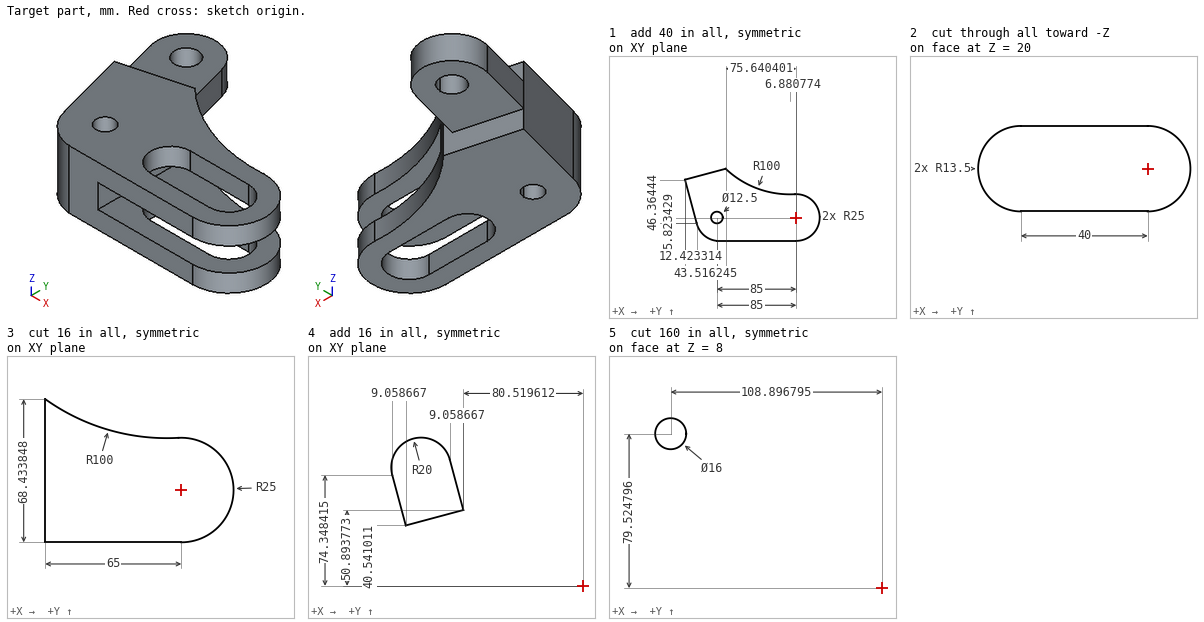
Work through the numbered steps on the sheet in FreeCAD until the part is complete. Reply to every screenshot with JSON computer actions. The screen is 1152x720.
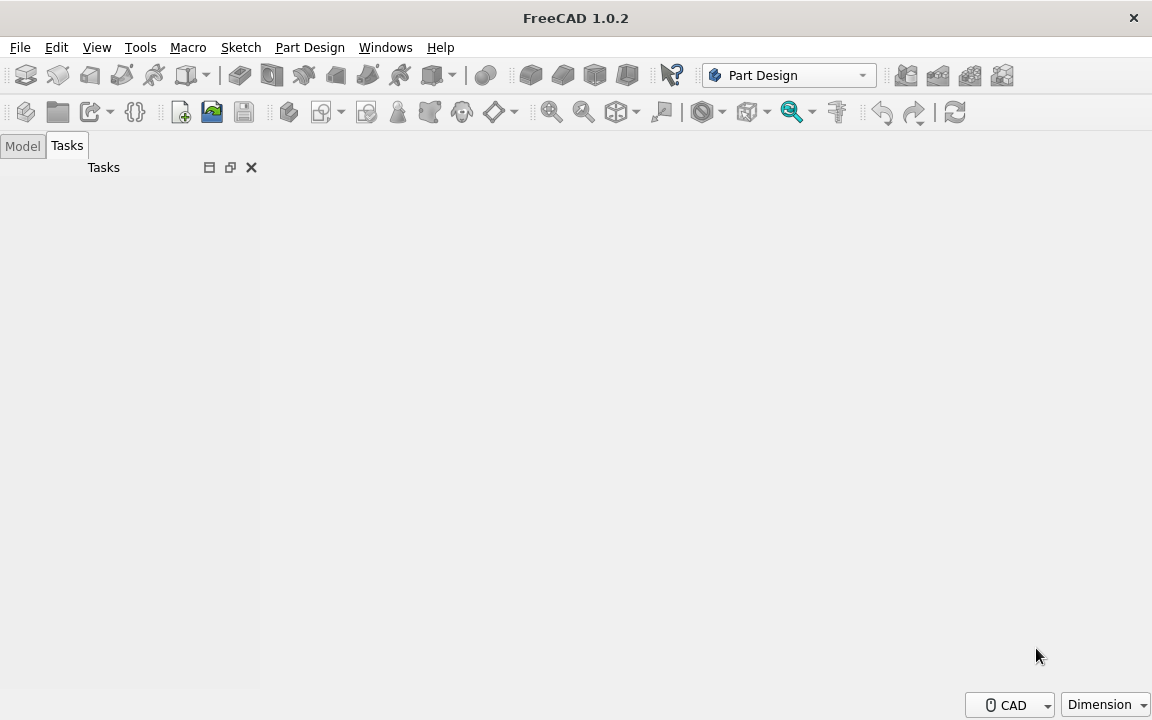
{"action": "left_click", "coordinate": [180, 112]}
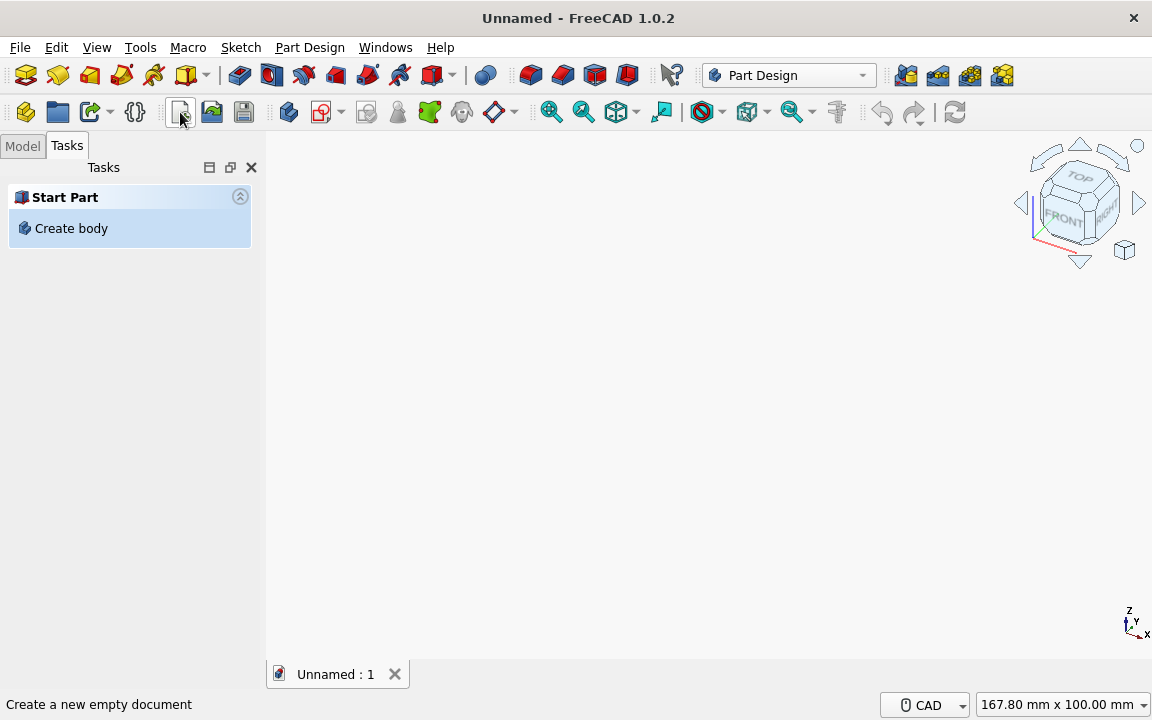
{"action": "left_click", "coordinate": [322, 112]}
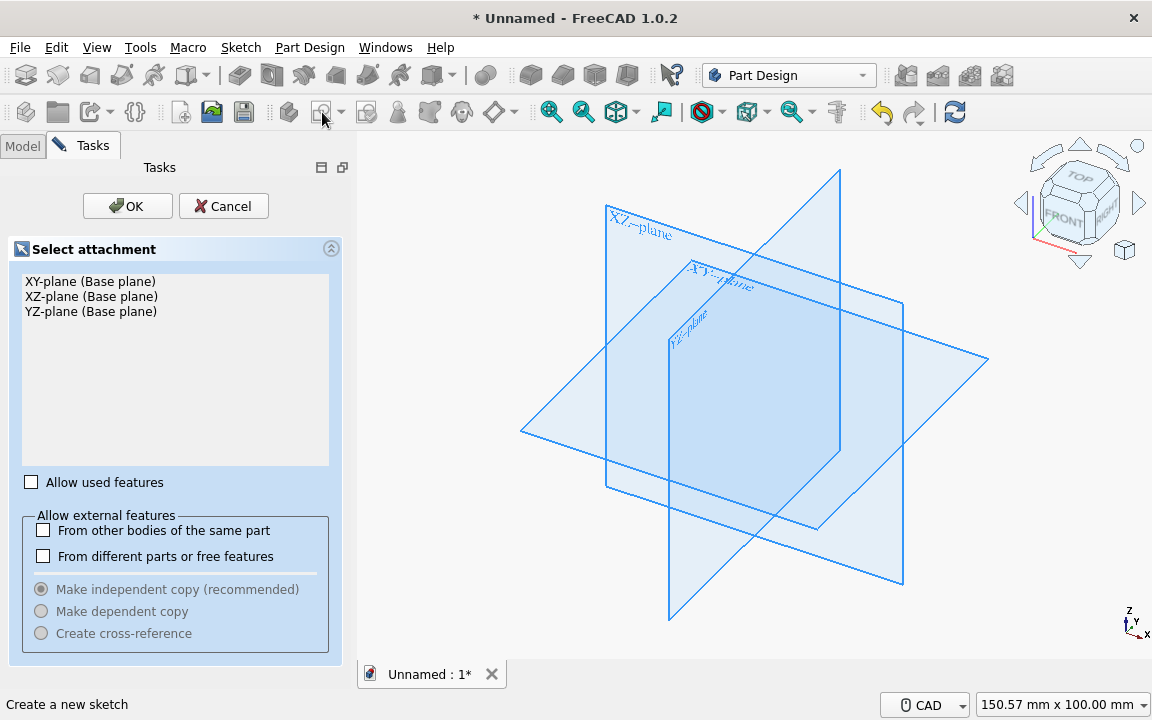
{"action": "left_click", "coordinate": [82, 282]}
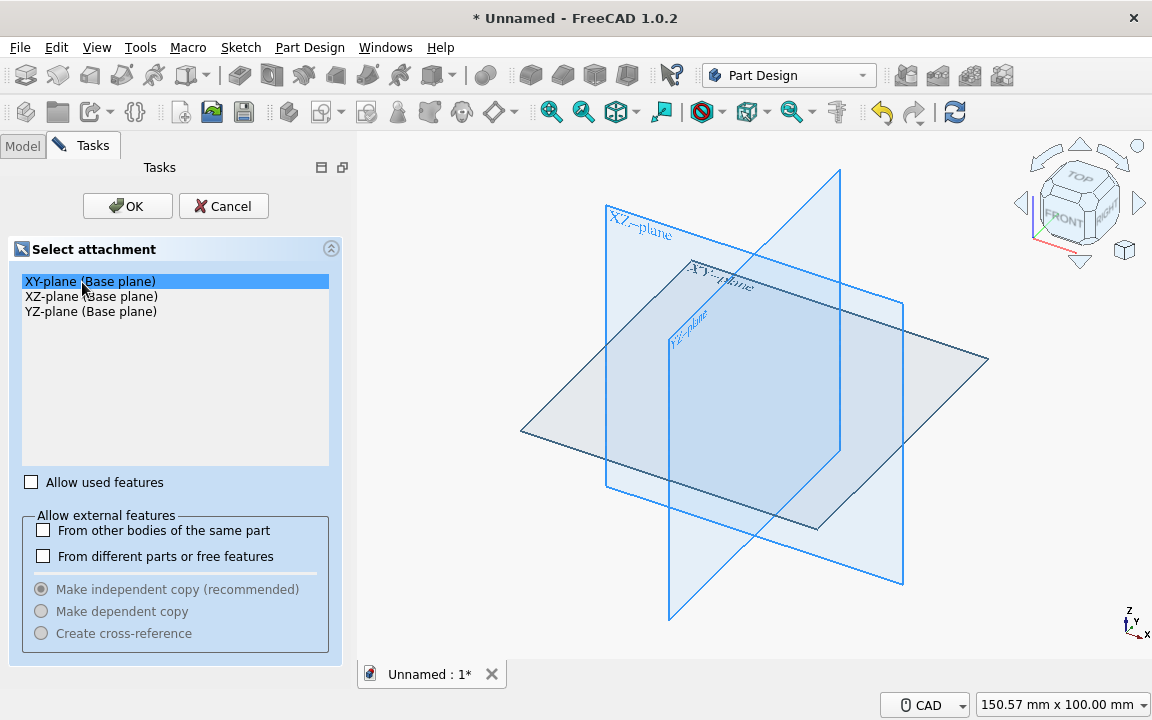
{"action": "left_click", "coordinate": [128, 206]}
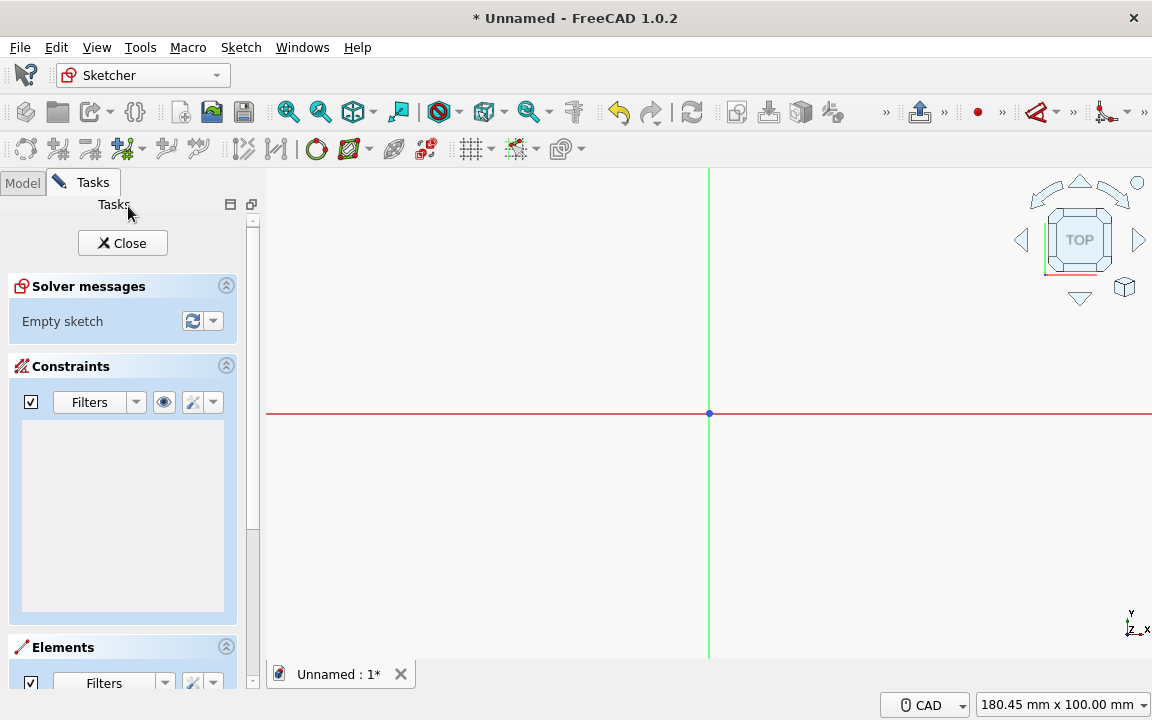
{"action": "scroll", "coordinate": [971, 549], "scroll_direction": "down", "scroll_amount": 2}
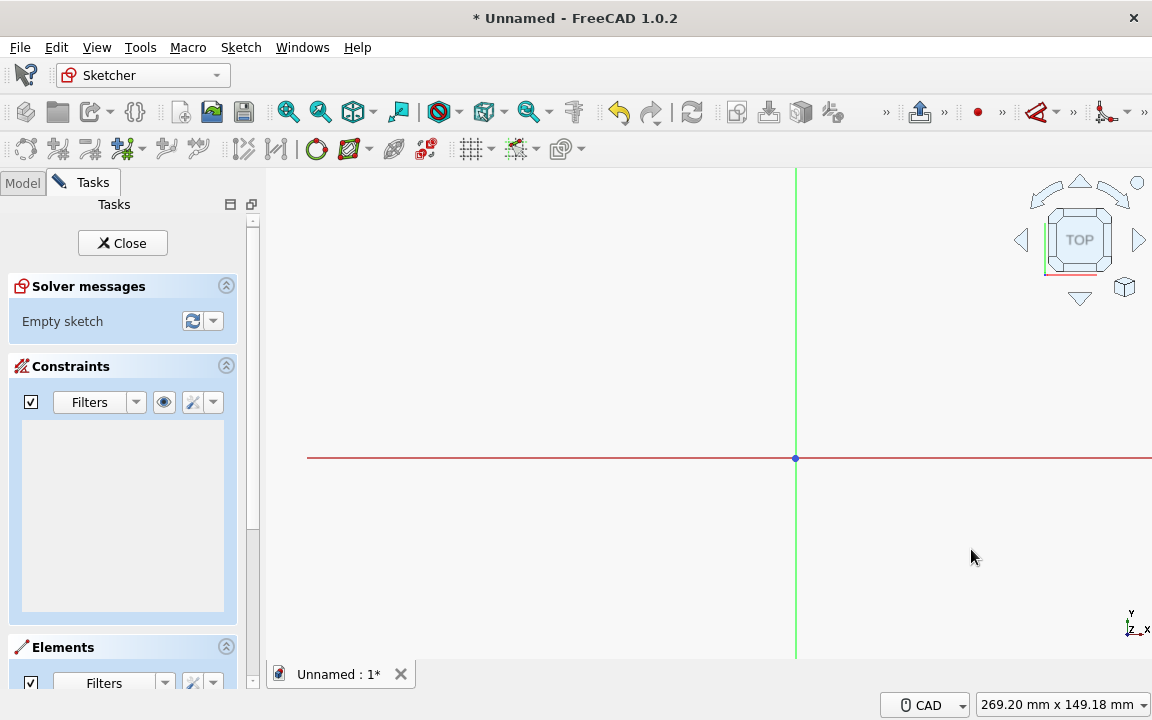
{"action": "key", "text": "g l"}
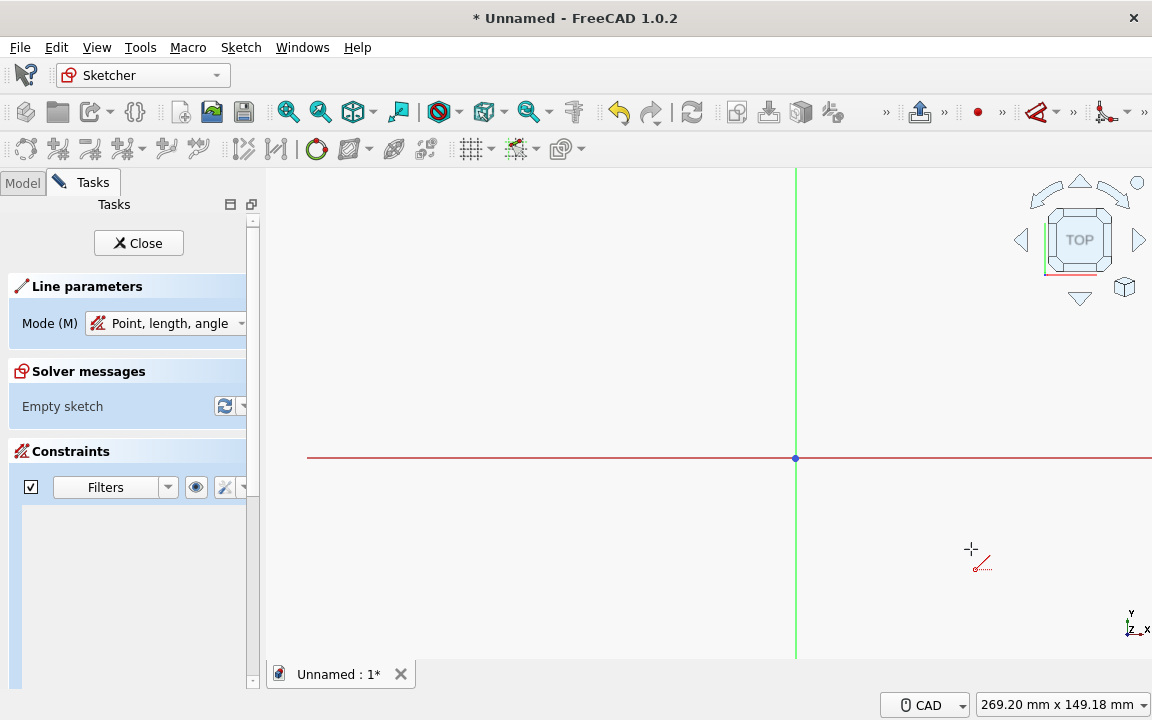
{"action": "left_click", "coordinate": [516, 541]}
{"action": "left_click", "coordinate": [796, 541]}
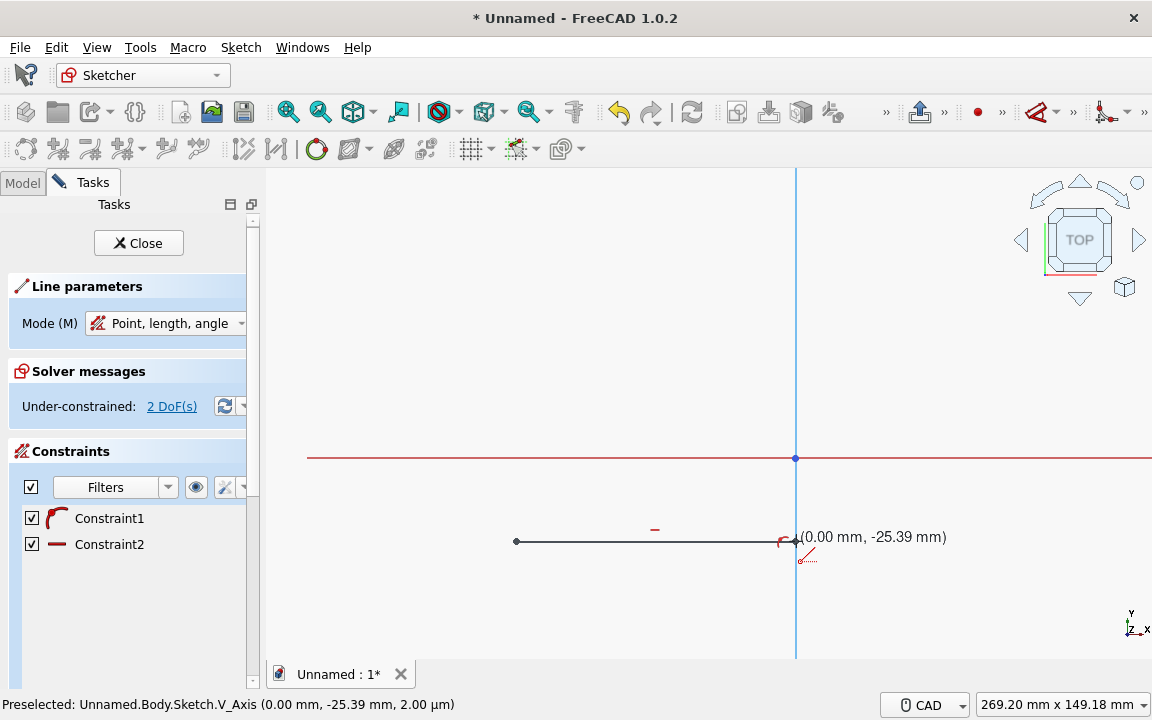
{"action": "key", "text": "g m"}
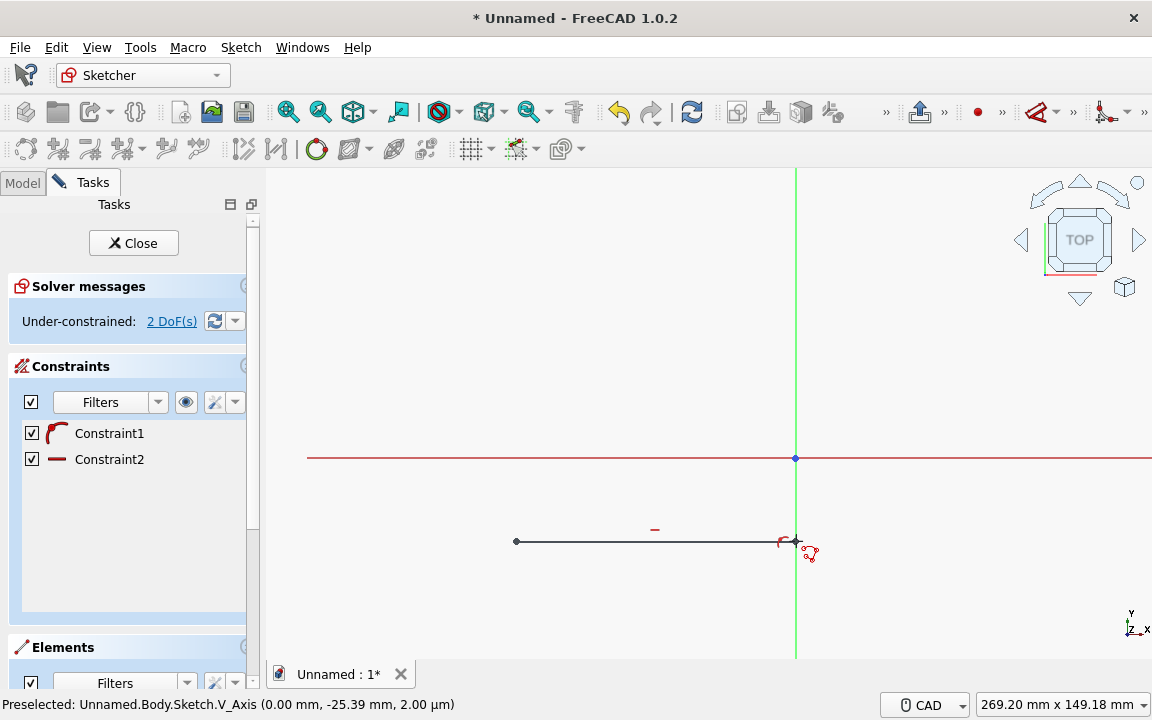
{"action": "left_click", "coordinate": [547, 287]}
{"action": "left_click", "coordinate": [403, 325]}
{"action": "left_click", "coordinate": [444, 478]}
{"action": "right_click", "coordinate": [444, 478]}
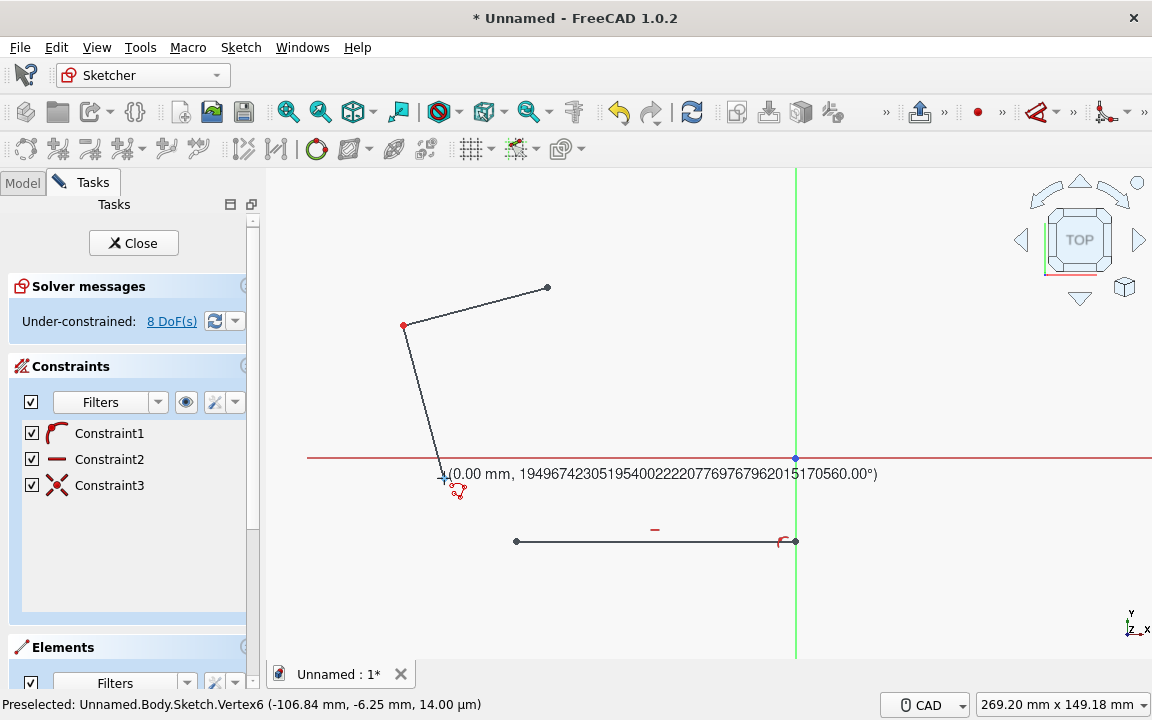
{"action": "key", "text": "g 3 a"}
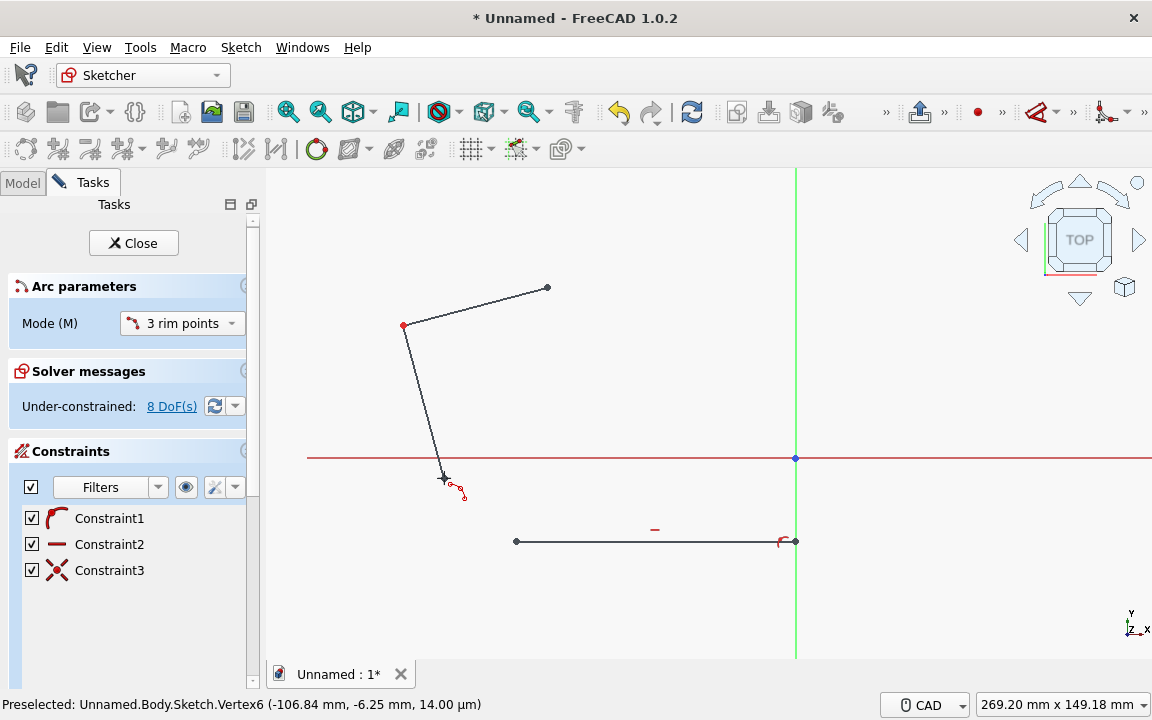
{"action": "left_click", "coordinate": [796, 542]}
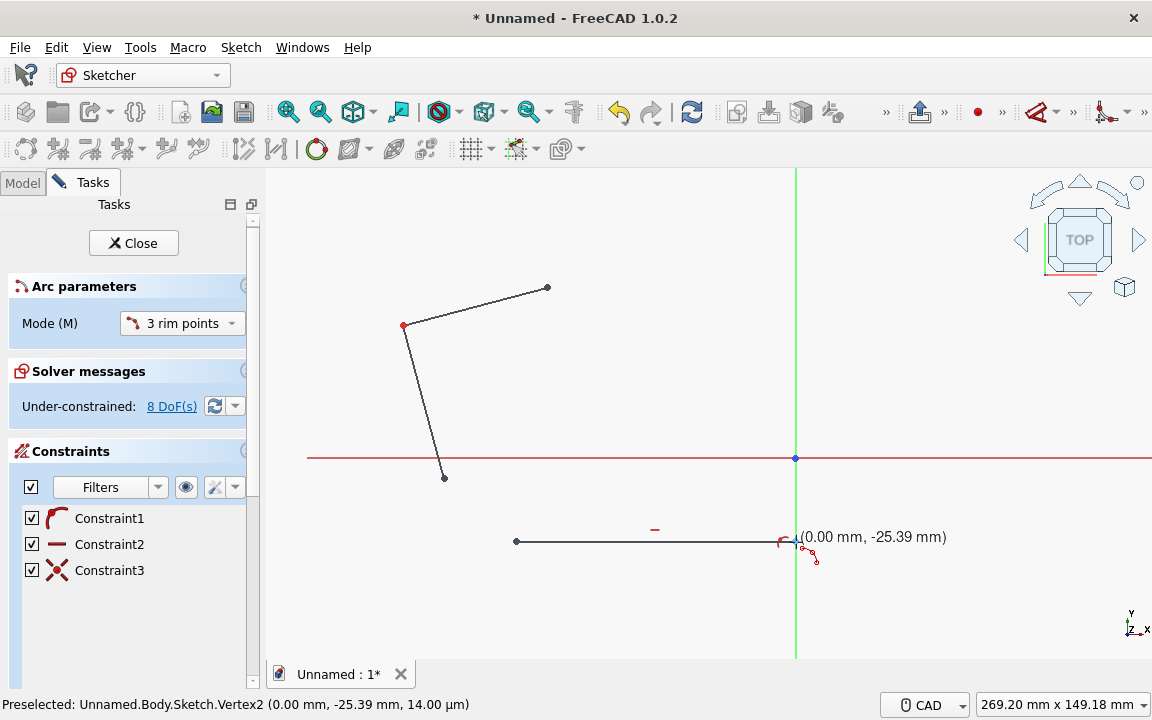
{"action": "scroll", "coordinate": [791, 376], "scroll_direction": "up", "scroll_amount": 7}